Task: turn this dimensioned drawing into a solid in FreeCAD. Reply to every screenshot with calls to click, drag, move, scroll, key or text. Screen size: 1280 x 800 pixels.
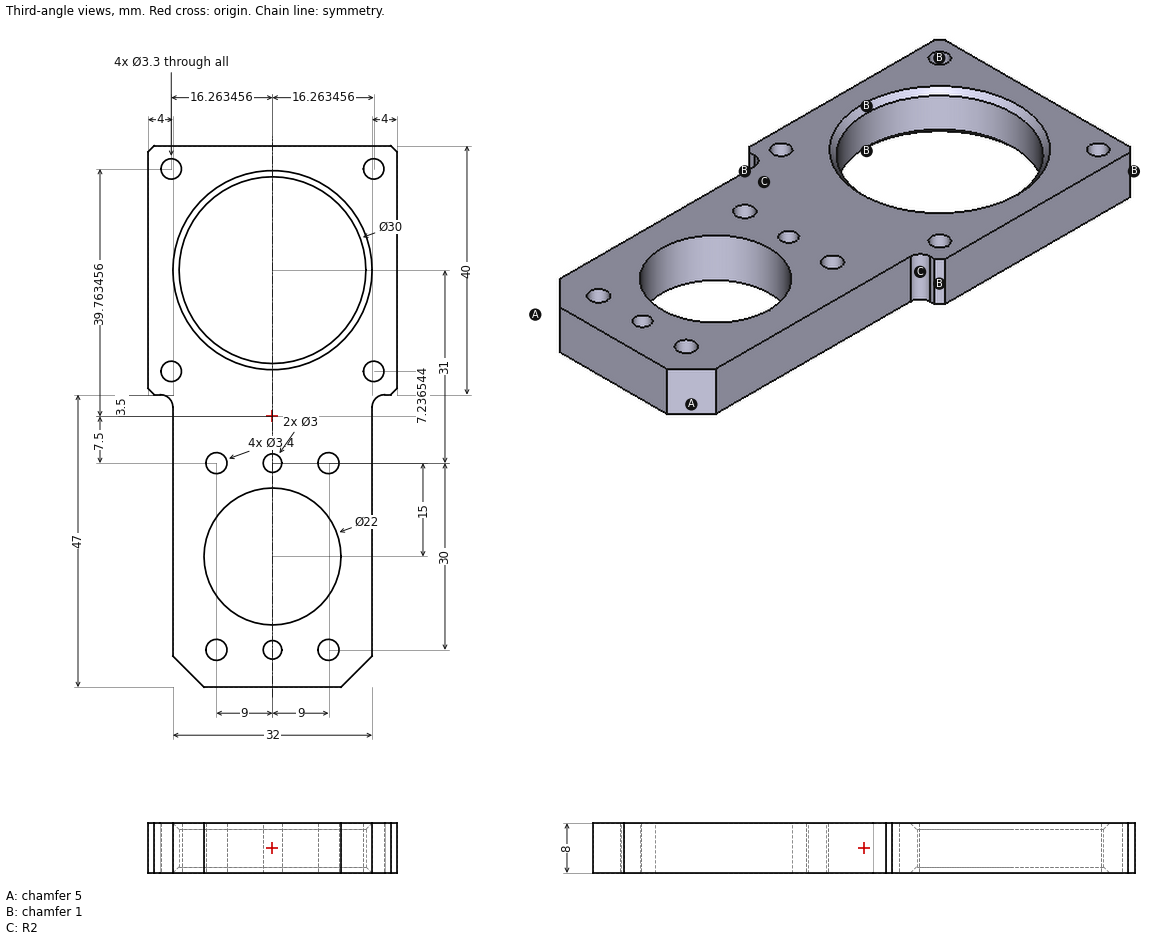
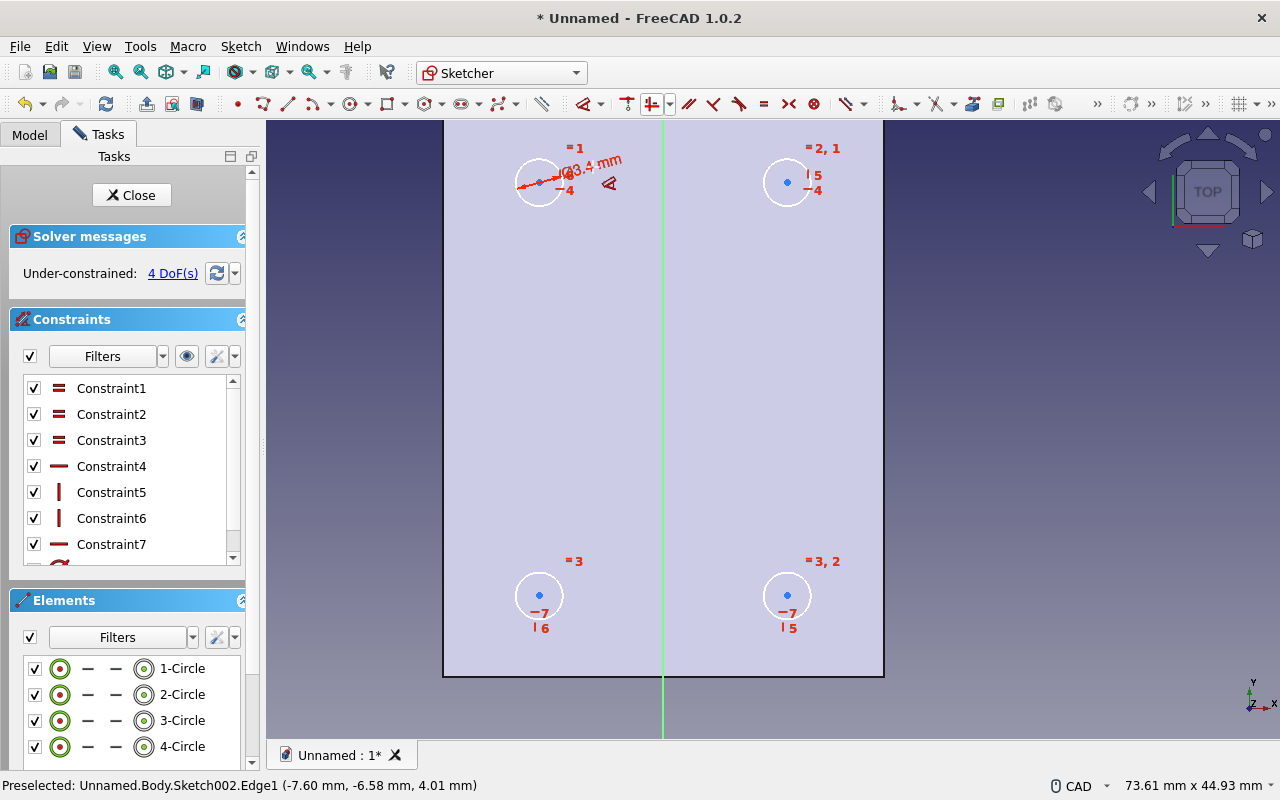
click(539, 183)
click(601, 217)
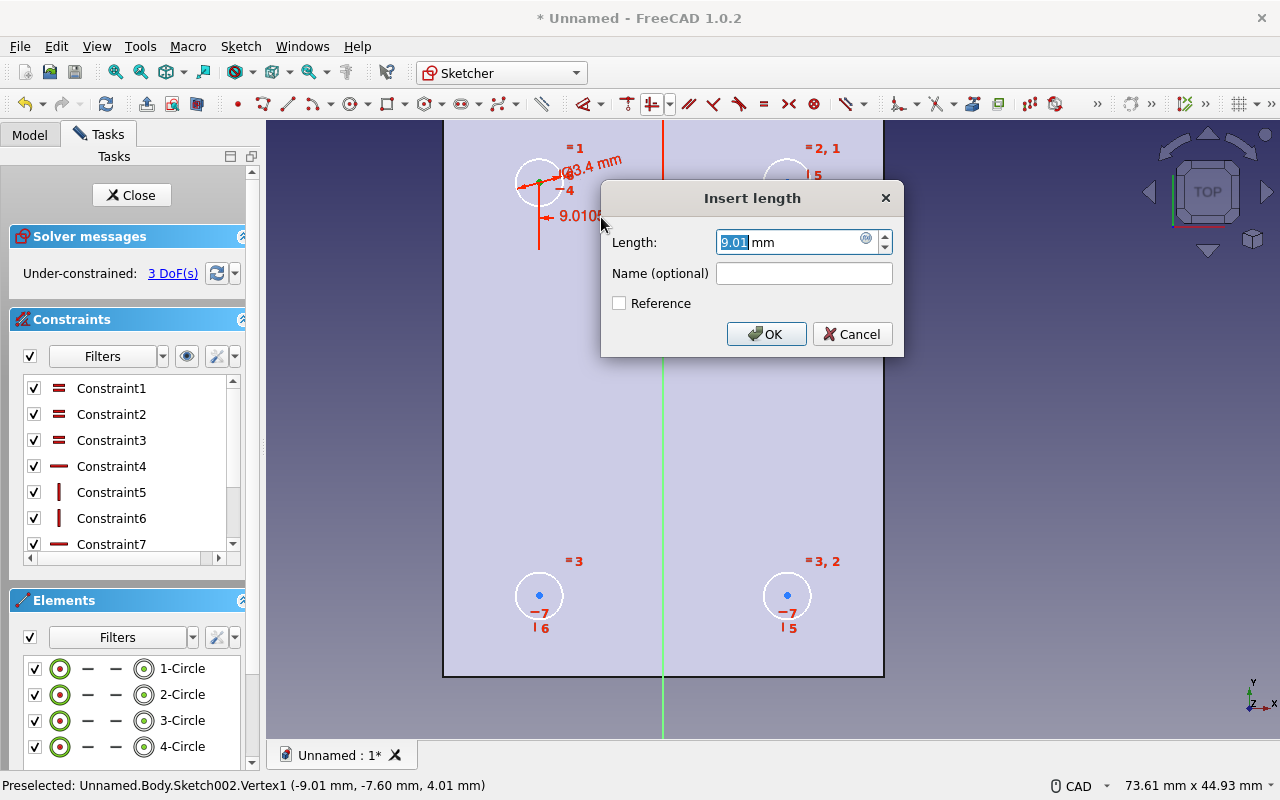
text(9)
key(Return)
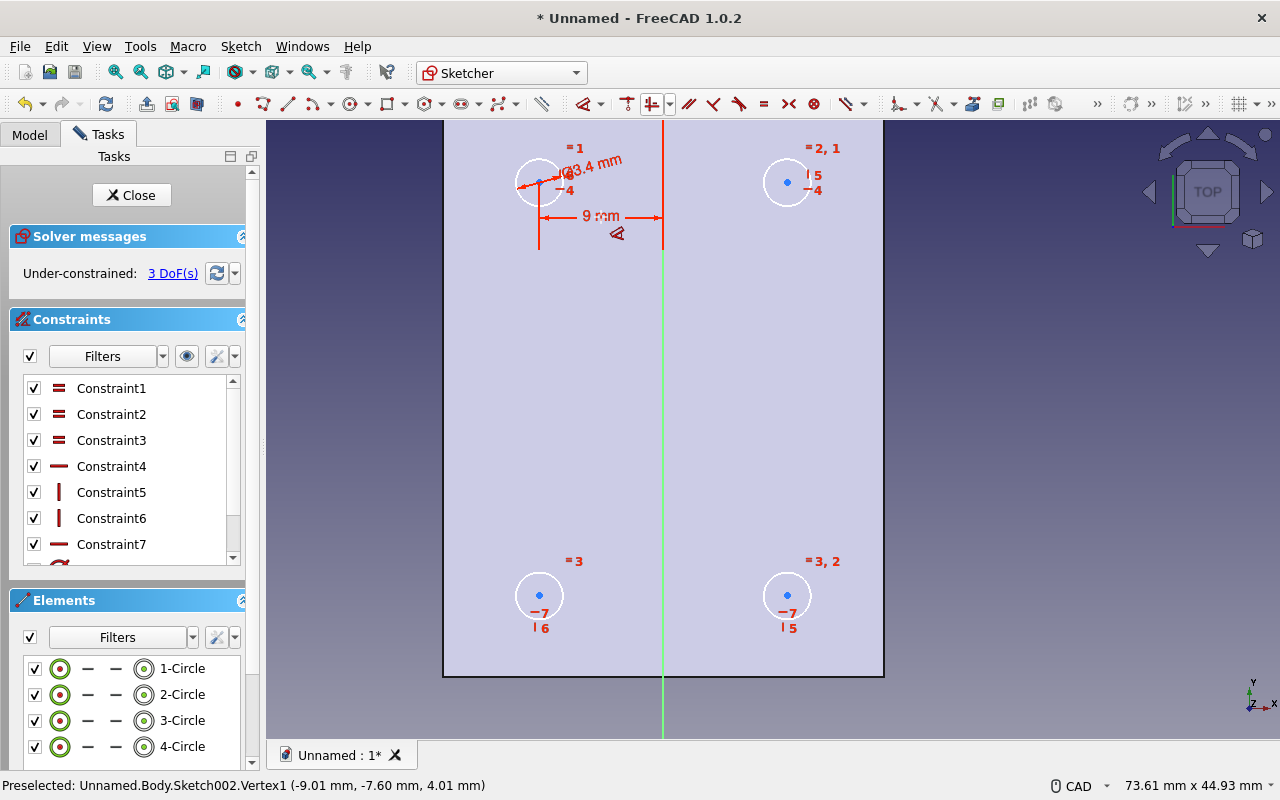
click(787, 183)
click(725, 217)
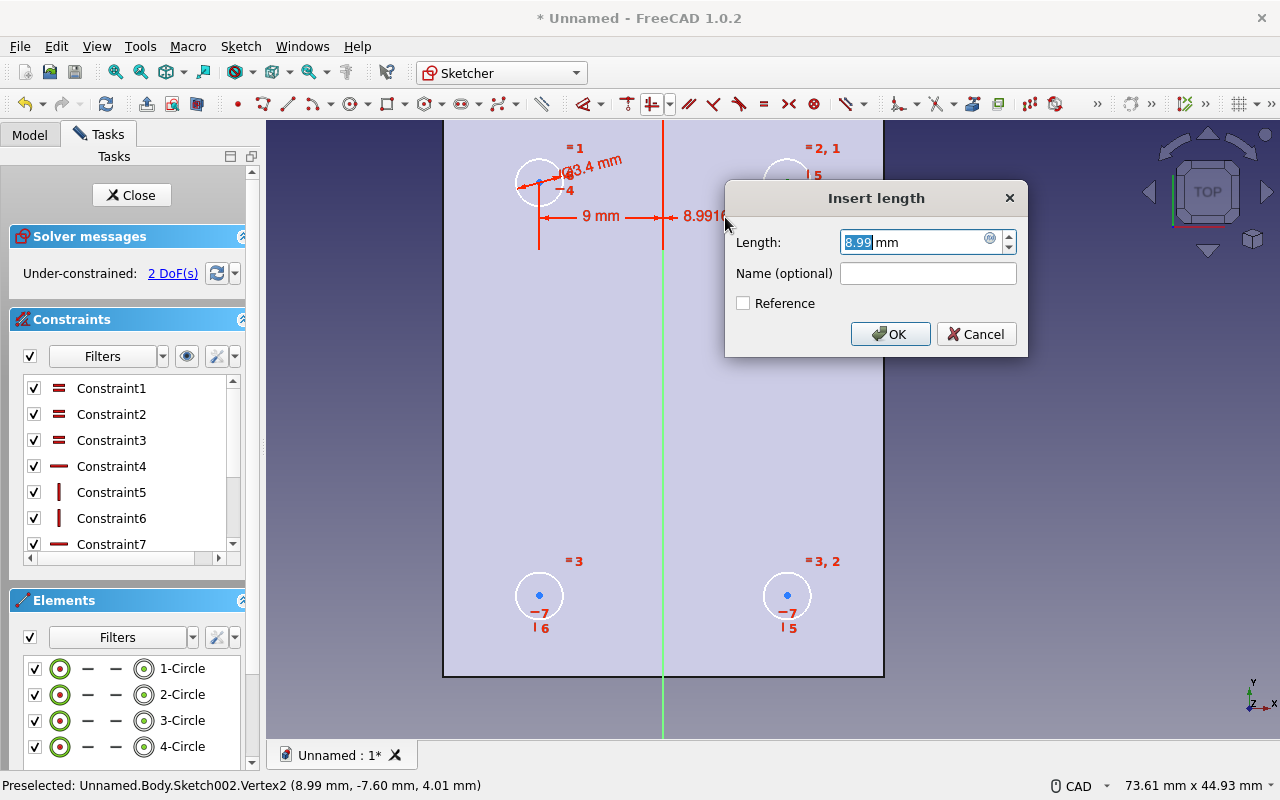
text(9)
key(Return)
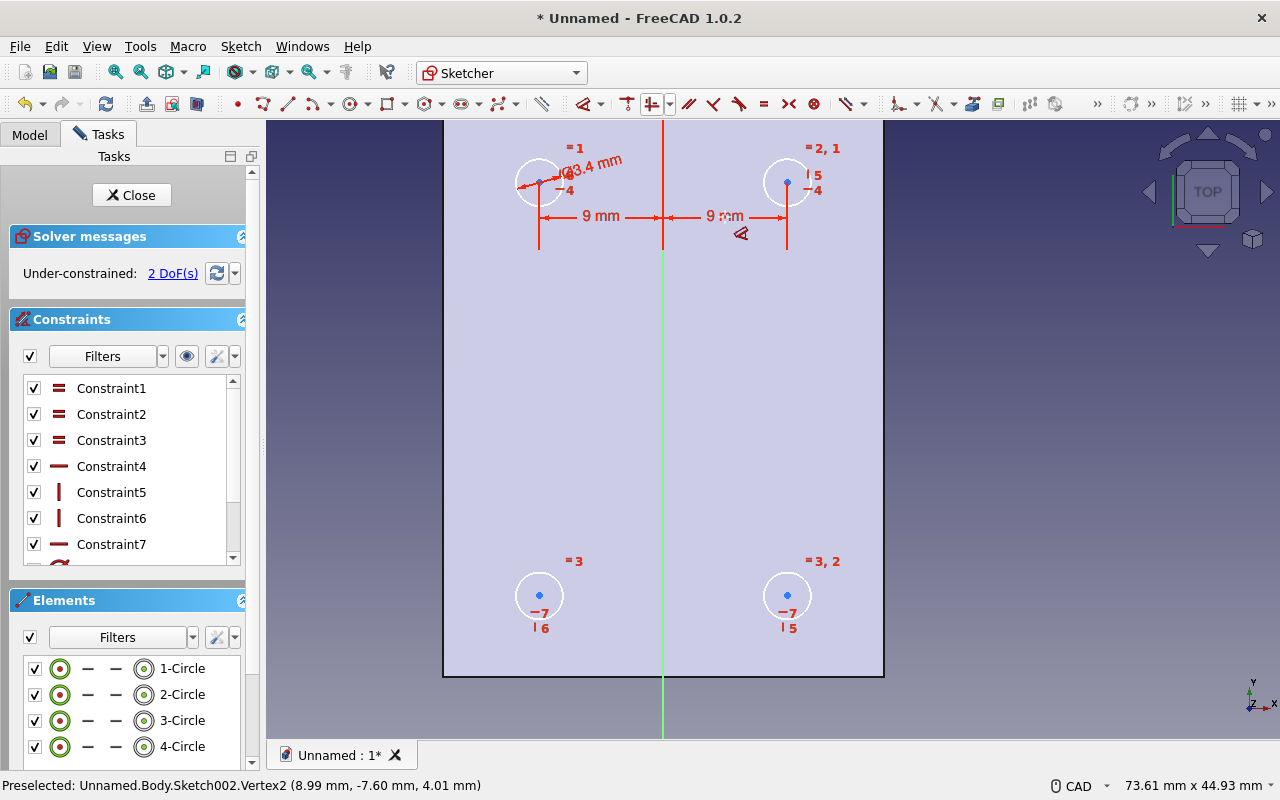
click(539, 183)
click(505, 165)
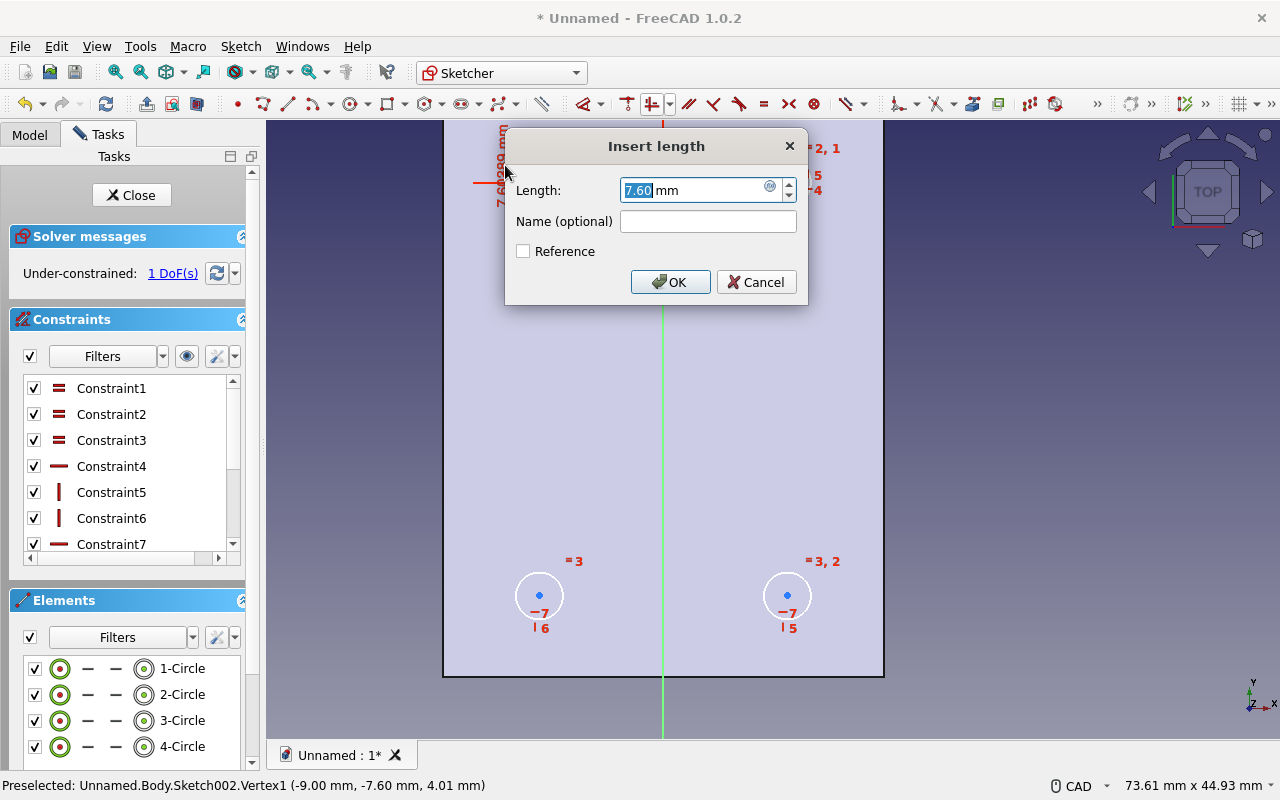
text(7.5)
key(Return)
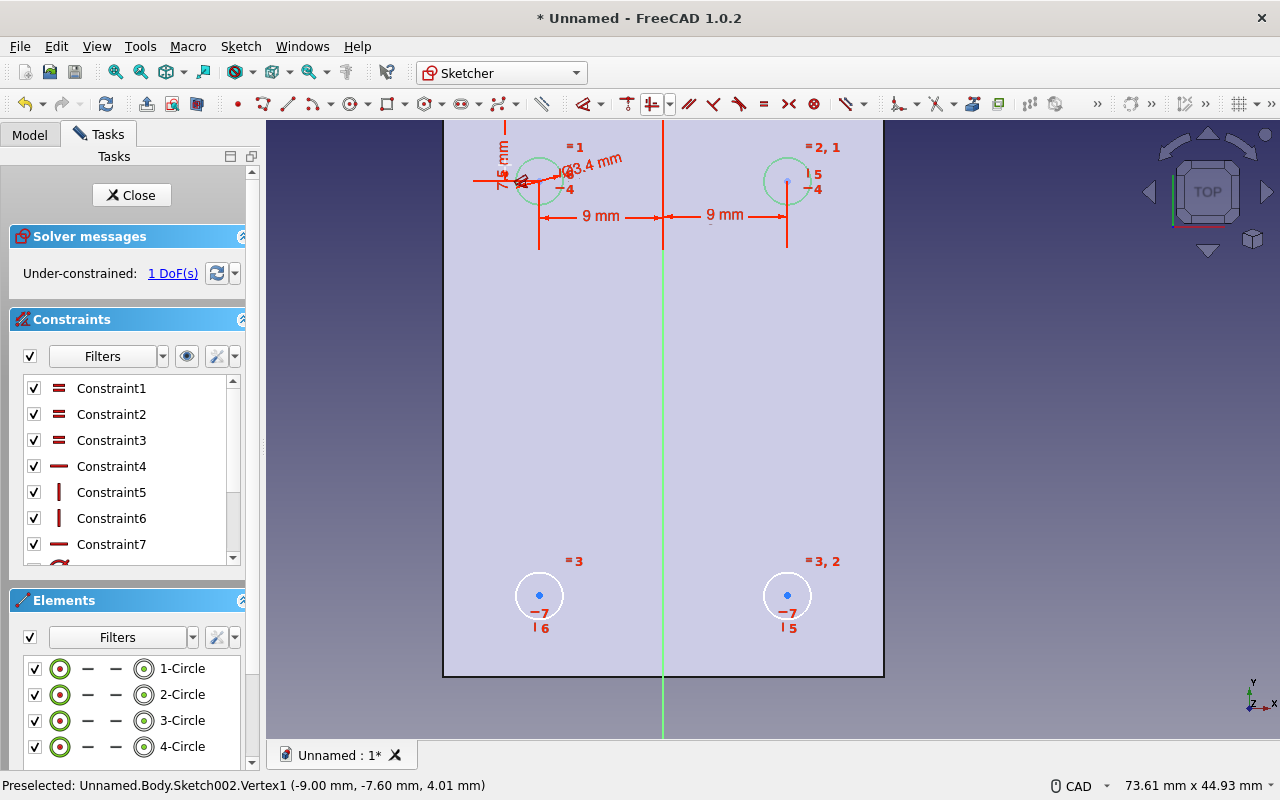
click(787, 181)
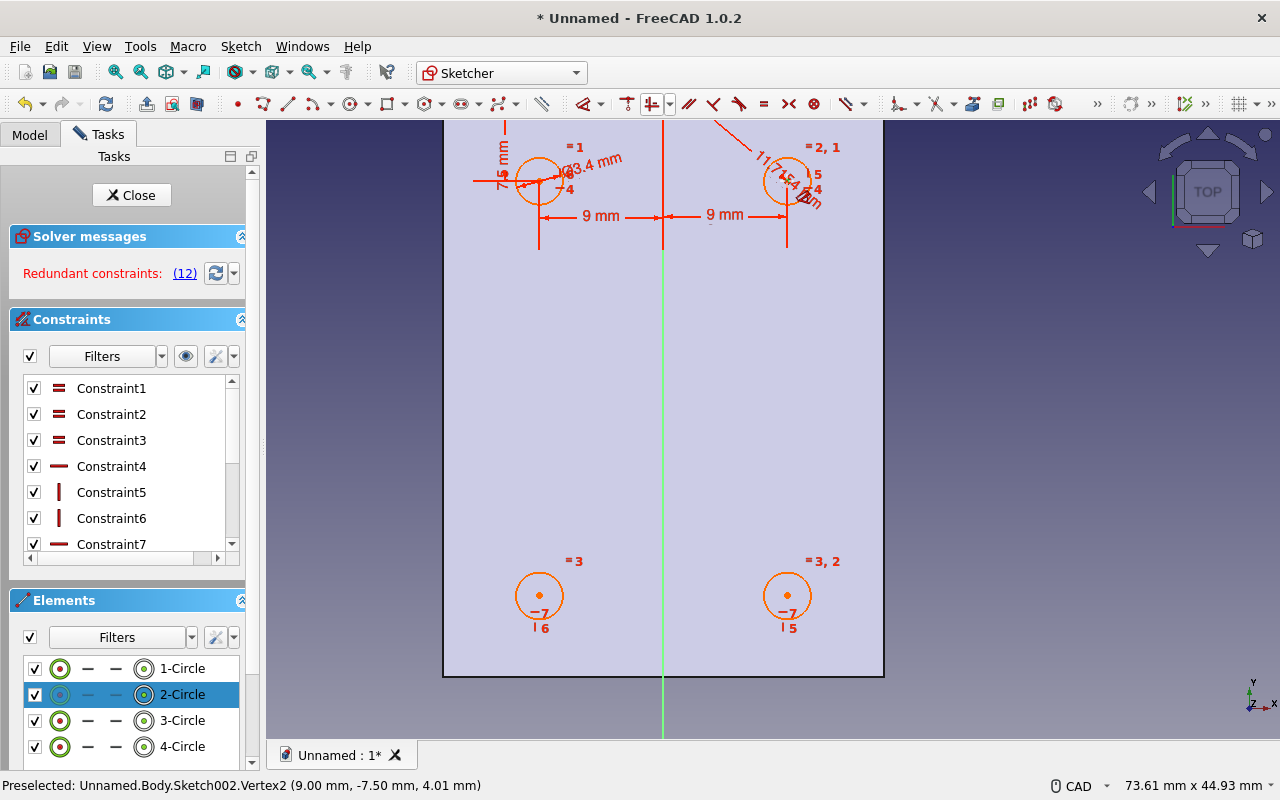
click(787, 596)
click(821, 389)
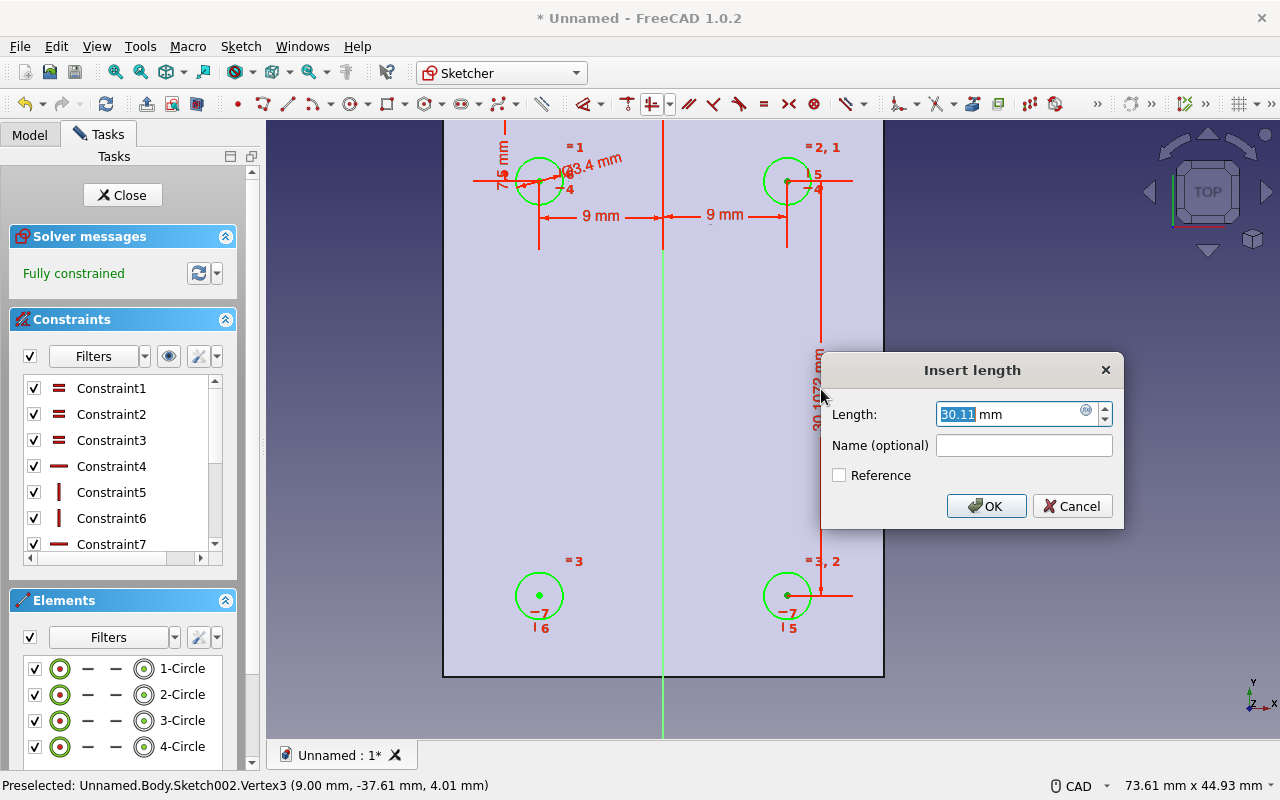
text(30)
key(Return)
key(Escape)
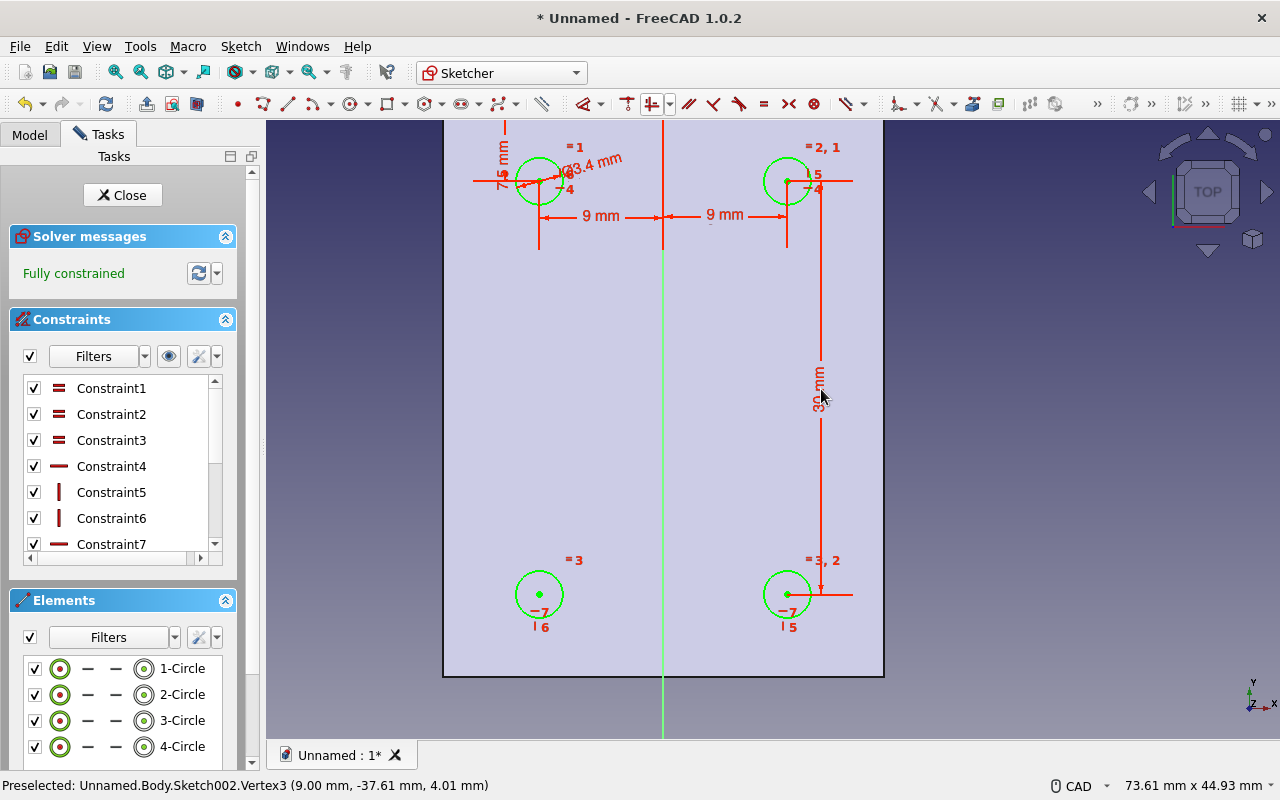
click(123, 195)